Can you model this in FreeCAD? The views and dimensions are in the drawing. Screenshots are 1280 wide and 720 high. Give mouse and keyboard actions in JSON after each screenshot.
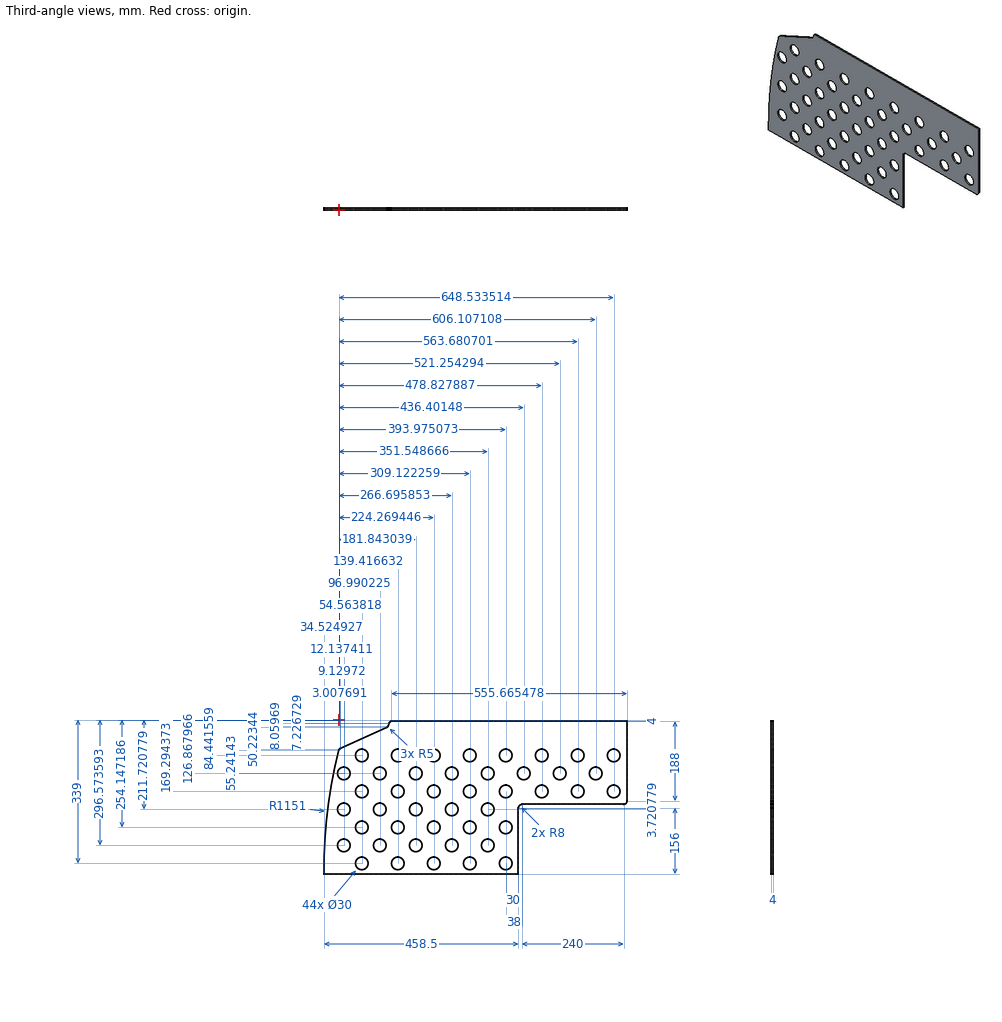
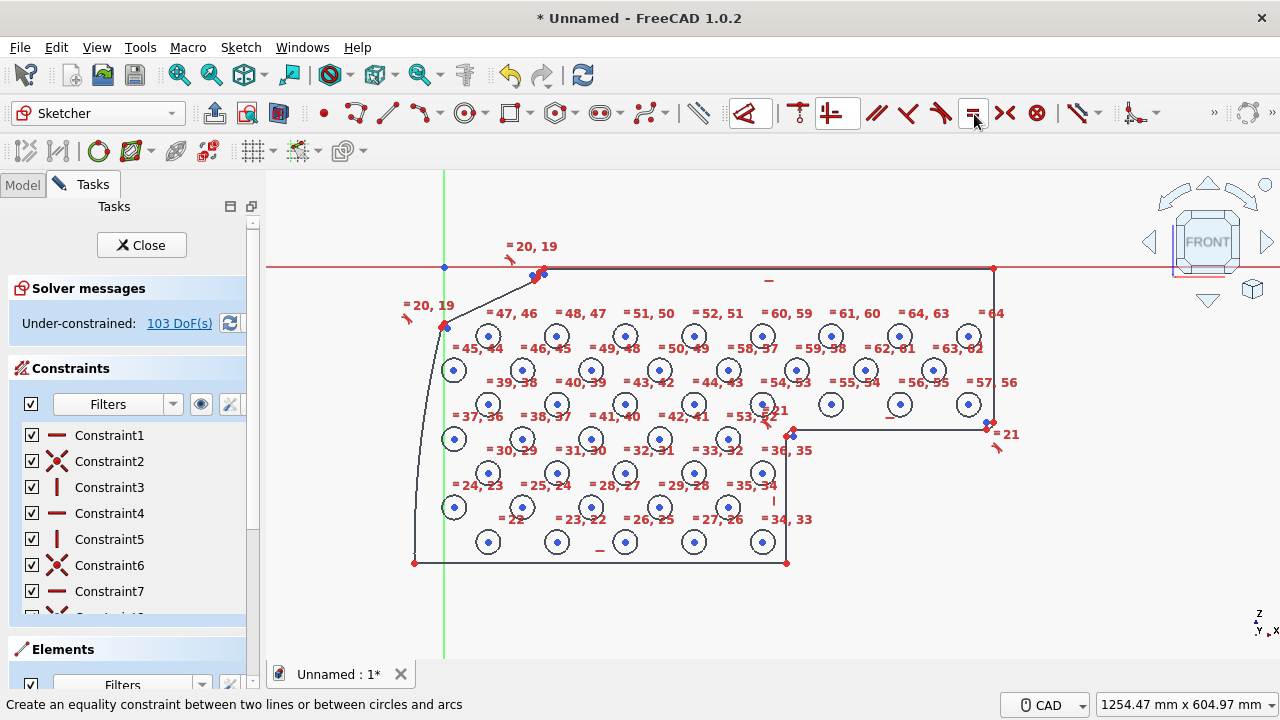
{"action": "key", "text": "d"}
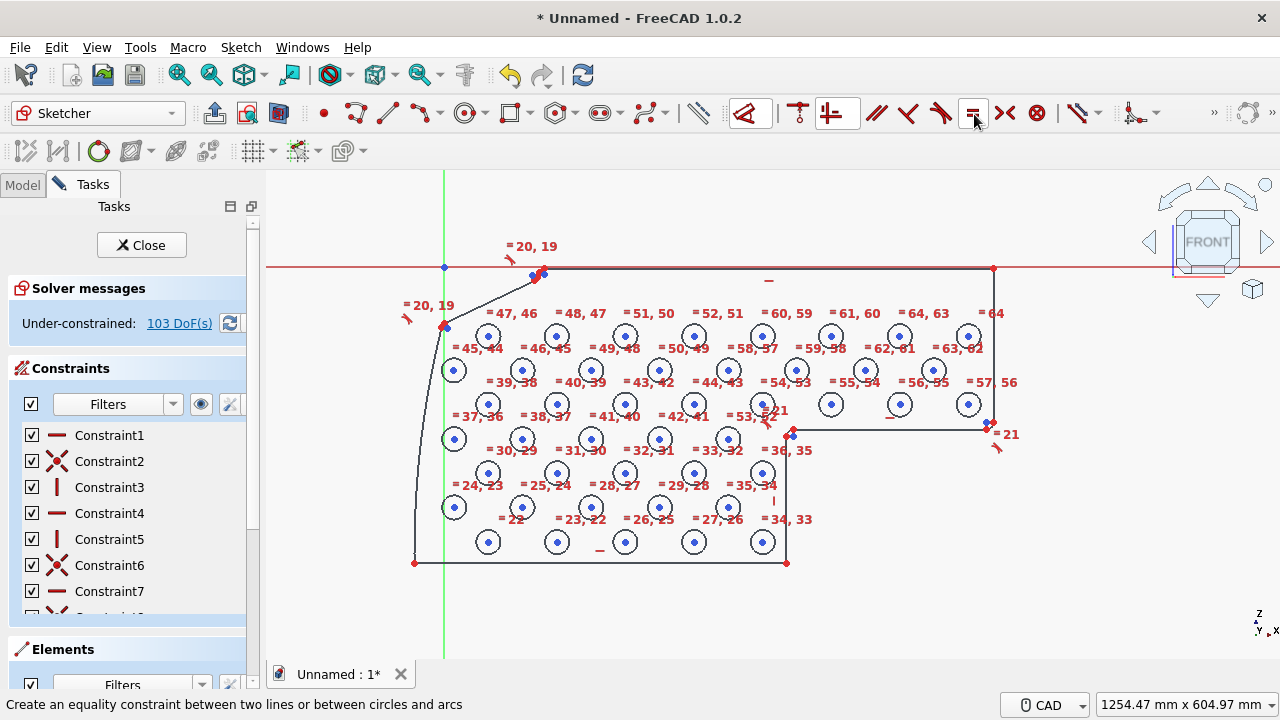
{"action": "scroll", "coordinate": [536, 280], "scroll_direction": "up", "scroll_amount": 12}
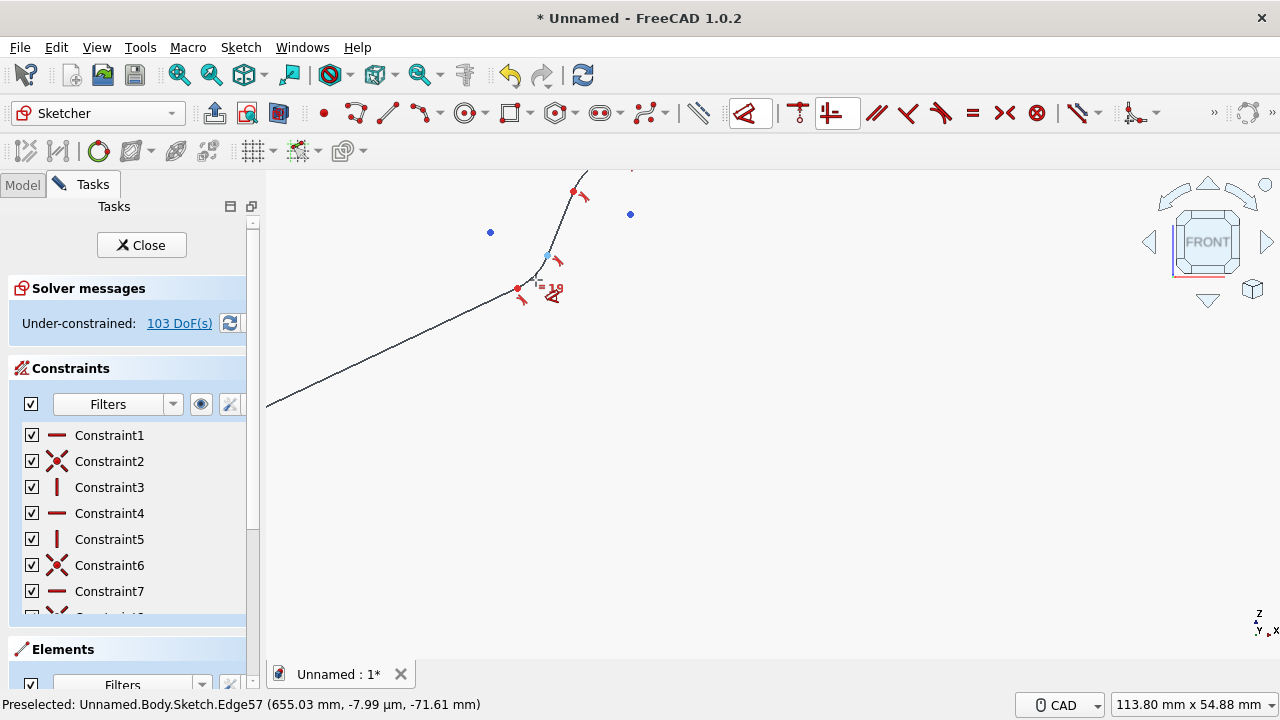
{"action": "left_click", "coordinate": [535, 275]}
{"action": "left_click", "coordinate": [558, 297]}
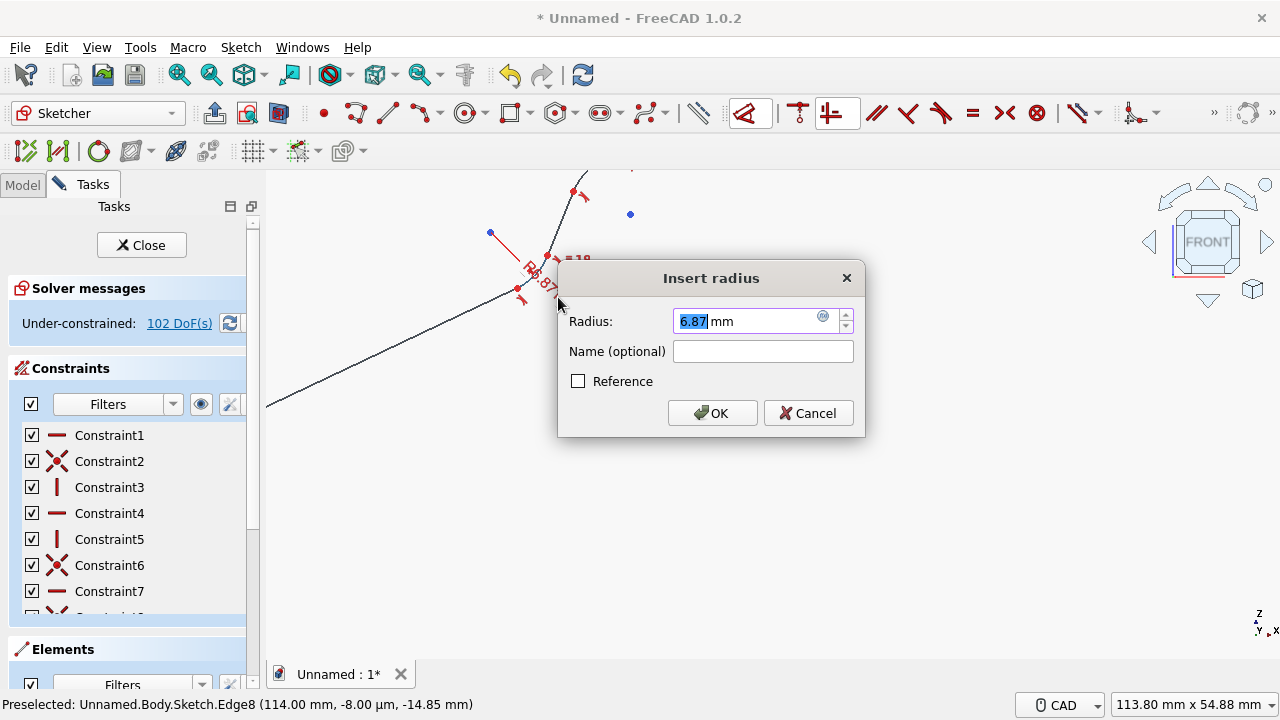
{"action": "type", "text": "5"}
{"action": "key", "text": "Return"}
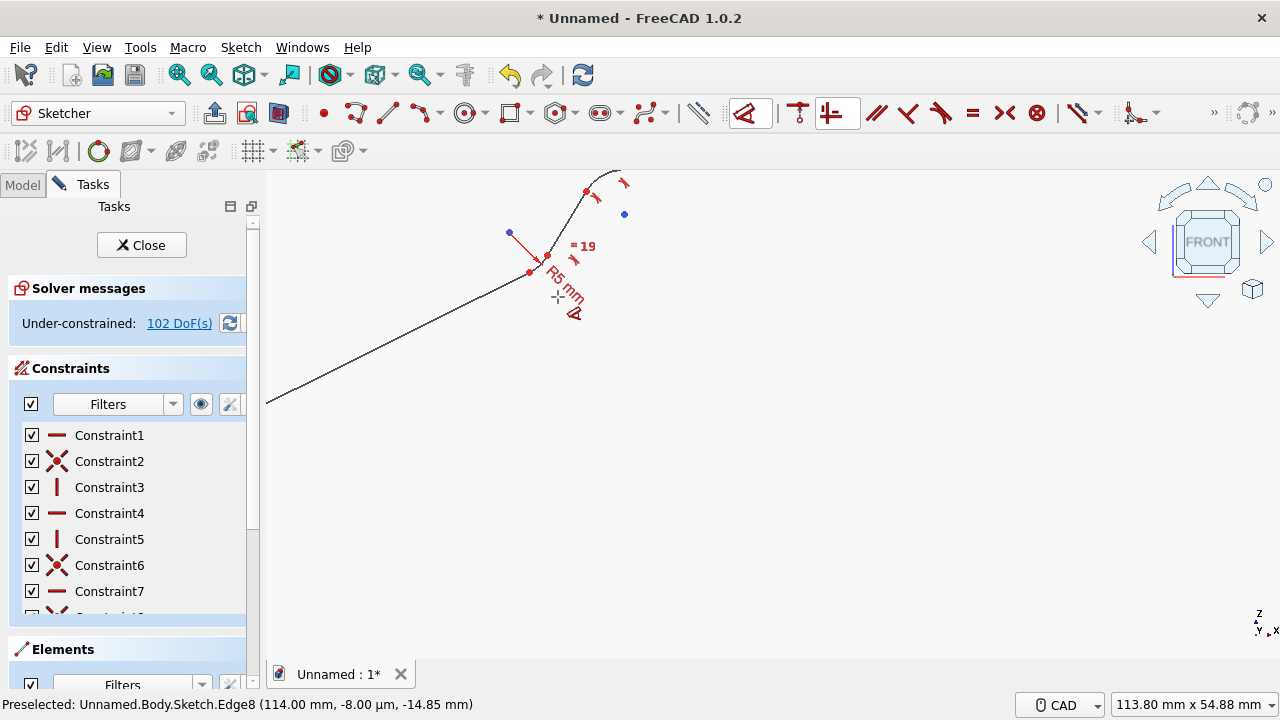
{"action": "scroll", "coordinate": [536, 280], "scroll_direction": "down", "scroll_amount": 12}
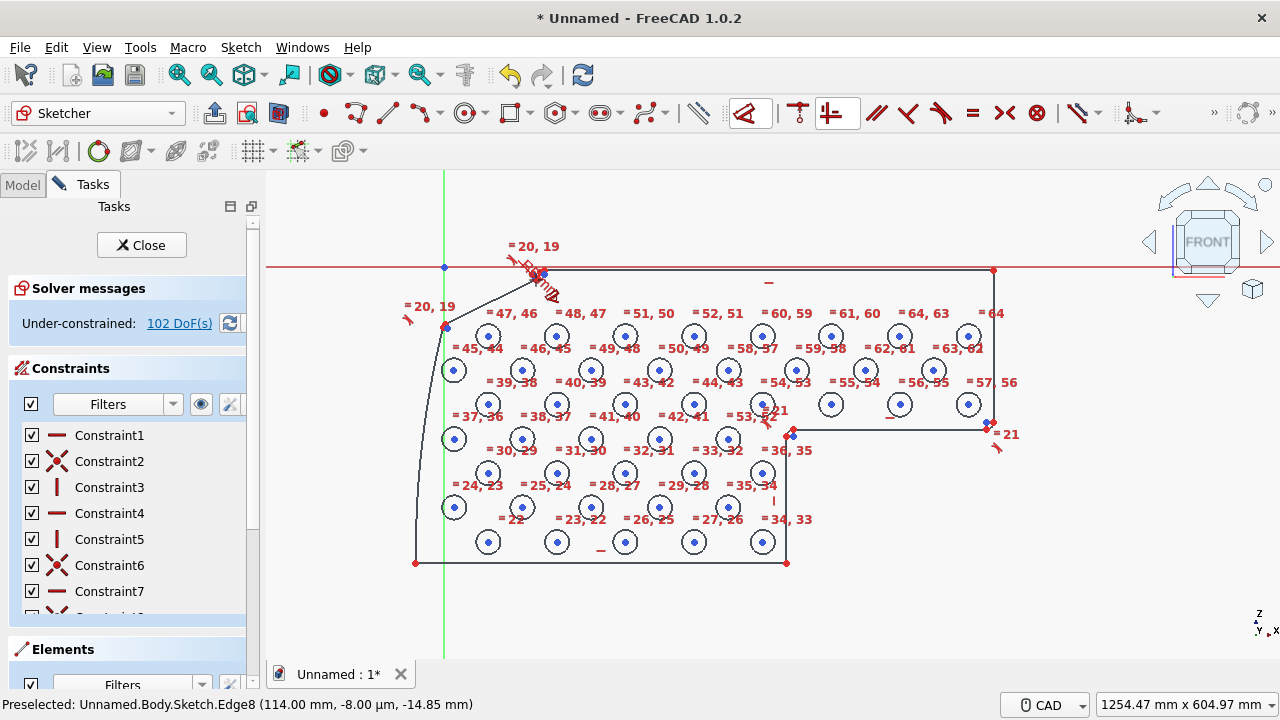
{"action": "left_click", "coordinate": [429, 397]}
{"action": "left_click", "coordinate": [397, 392]}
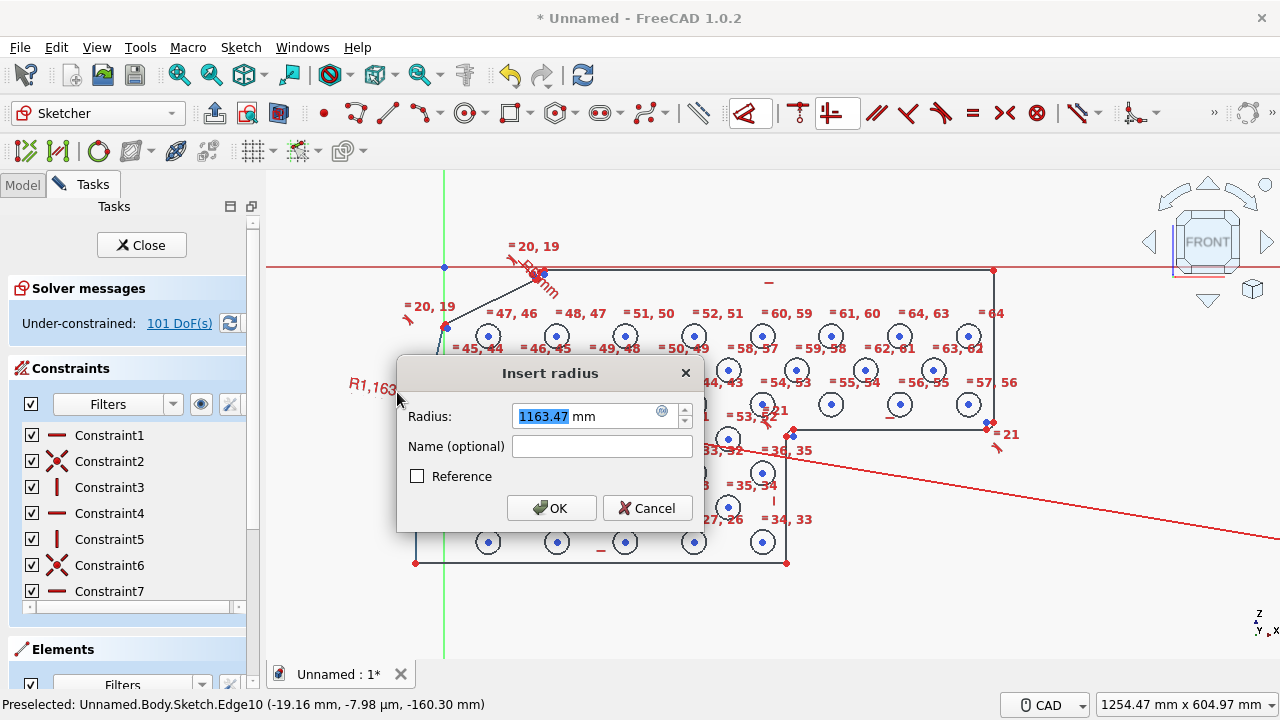
{"action": "type", "text": "1151"}
{"action": "key", "text": "Return"}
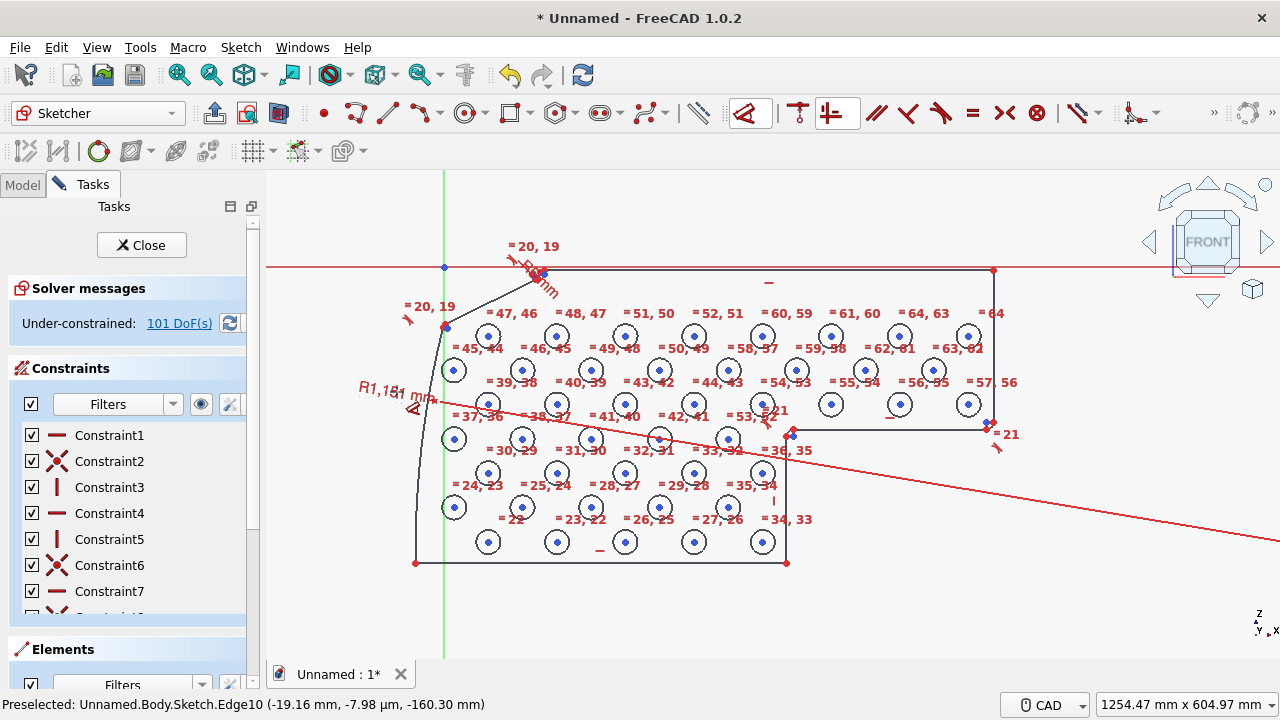
{"action": "scroll", "coordinate": [788, 432], "scroll_direction": "up", "scroll_amount": 10}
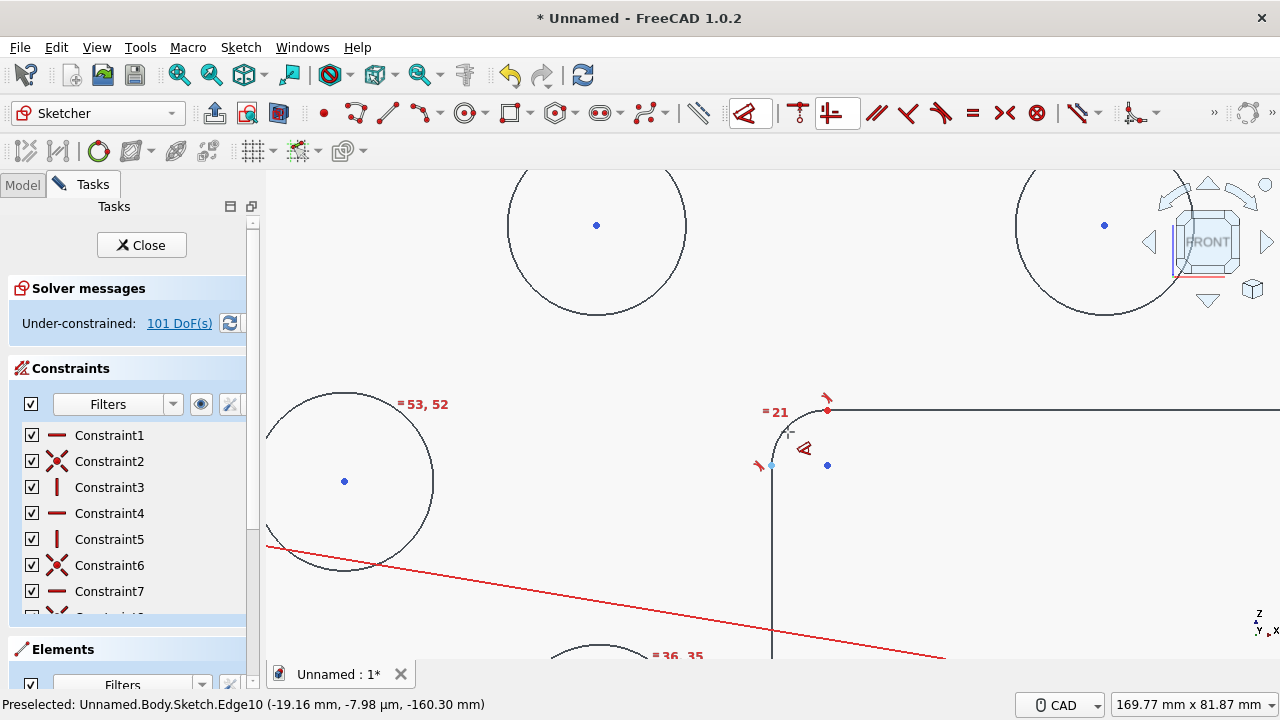
{"action": "left_click", "coordinate": [788, 426]}
{"action": "left_click", "coordinate": [765, 403]}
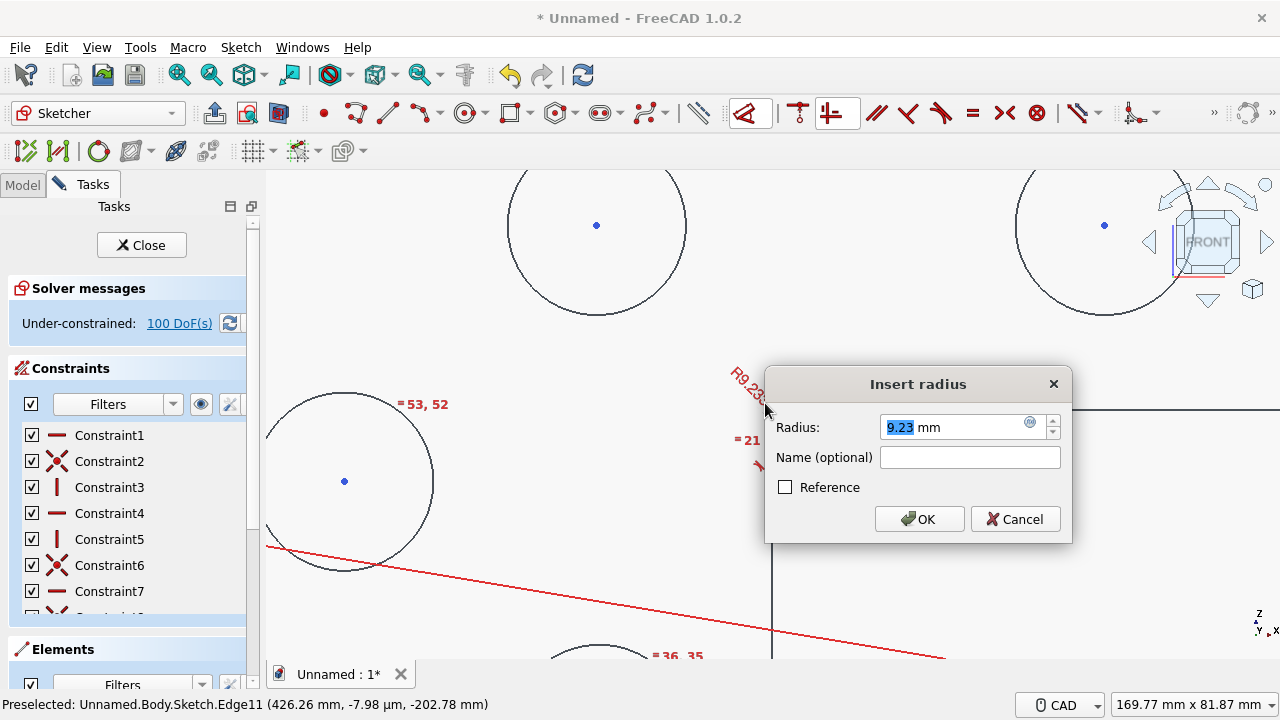
{"action": "type", "text": "8"}
{"action": "key", "text": "Return"}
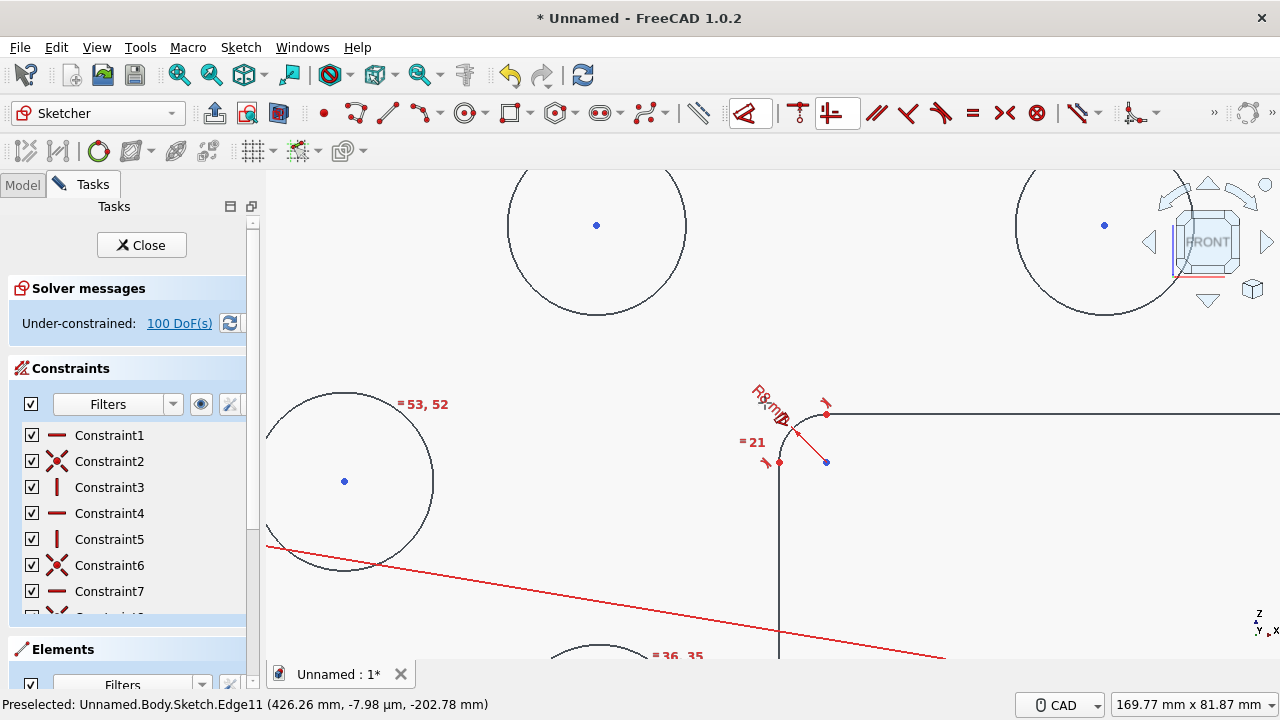
{"action": "scroll", "coordinate": [788, 432], "scroll_direction": "down", "scroll_amount": 10}